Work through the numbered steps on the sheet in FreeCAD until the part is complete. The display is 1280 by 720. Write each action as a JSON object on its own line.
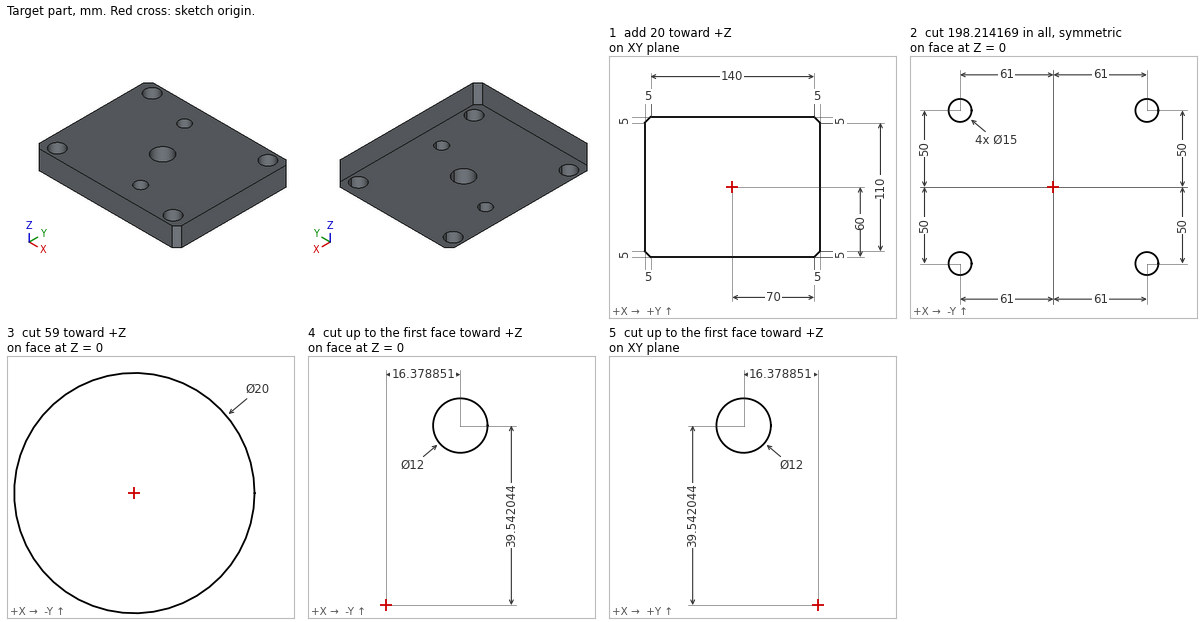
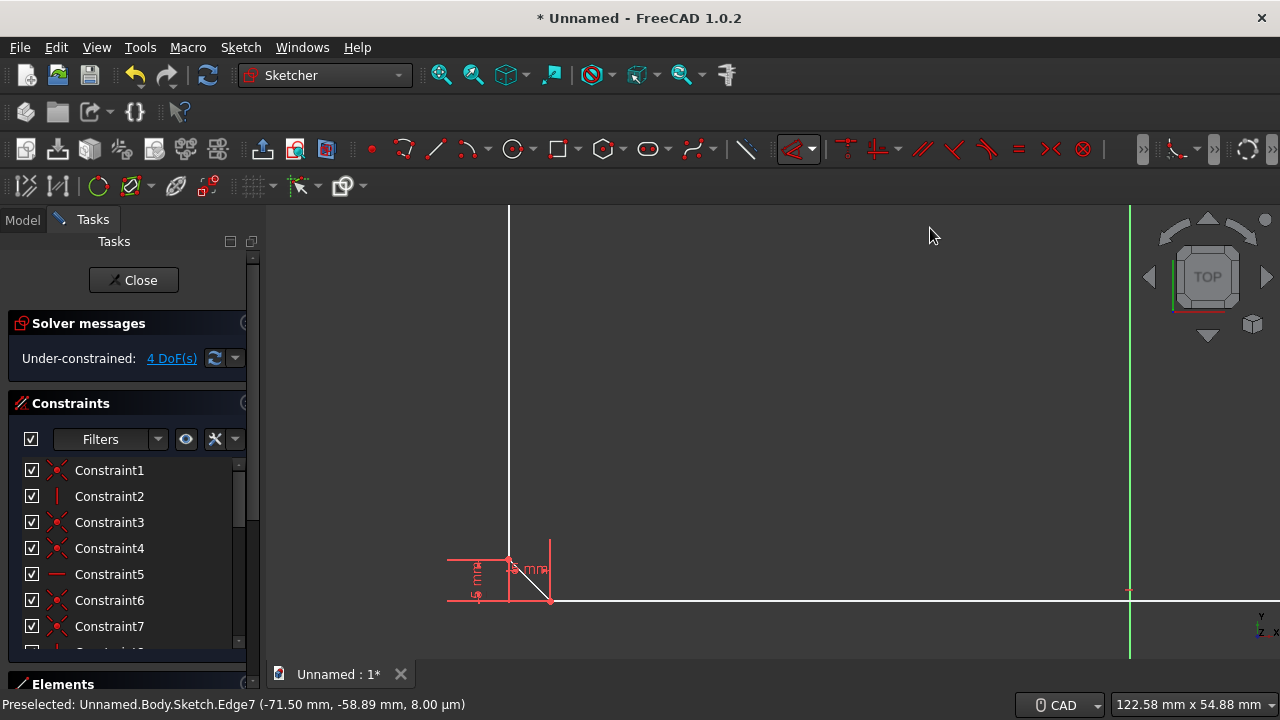
{"action": "scroll", "coordinate": [521, 574], "scroll_direction": "down", "scroll_amount": 6}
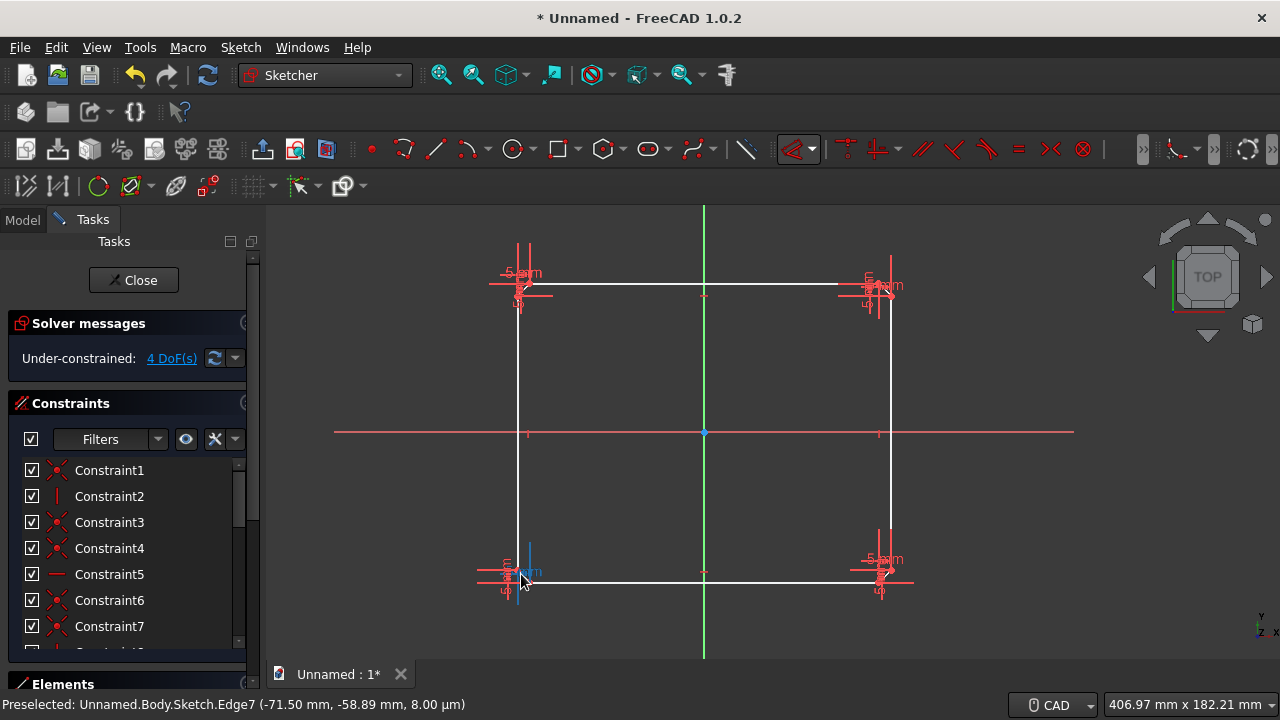
{"action": "left_click", "coordinate": [891, 488]}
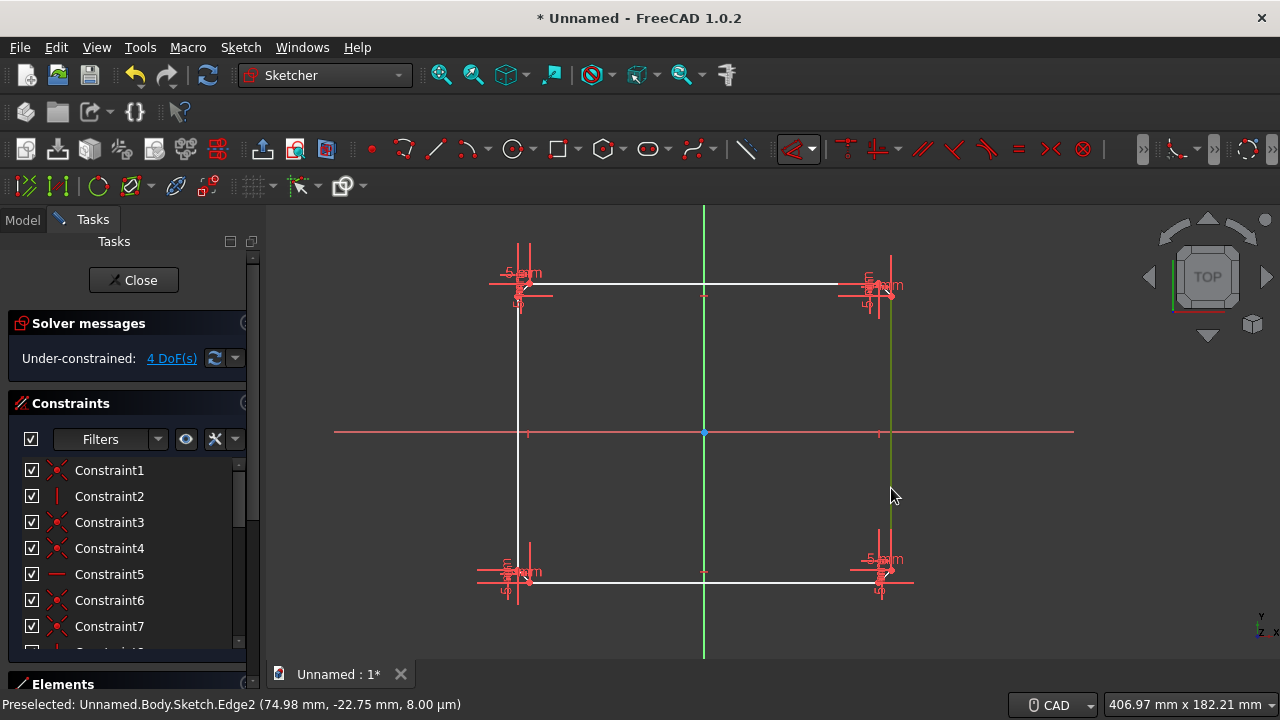
{"action": "key", "text": "i"}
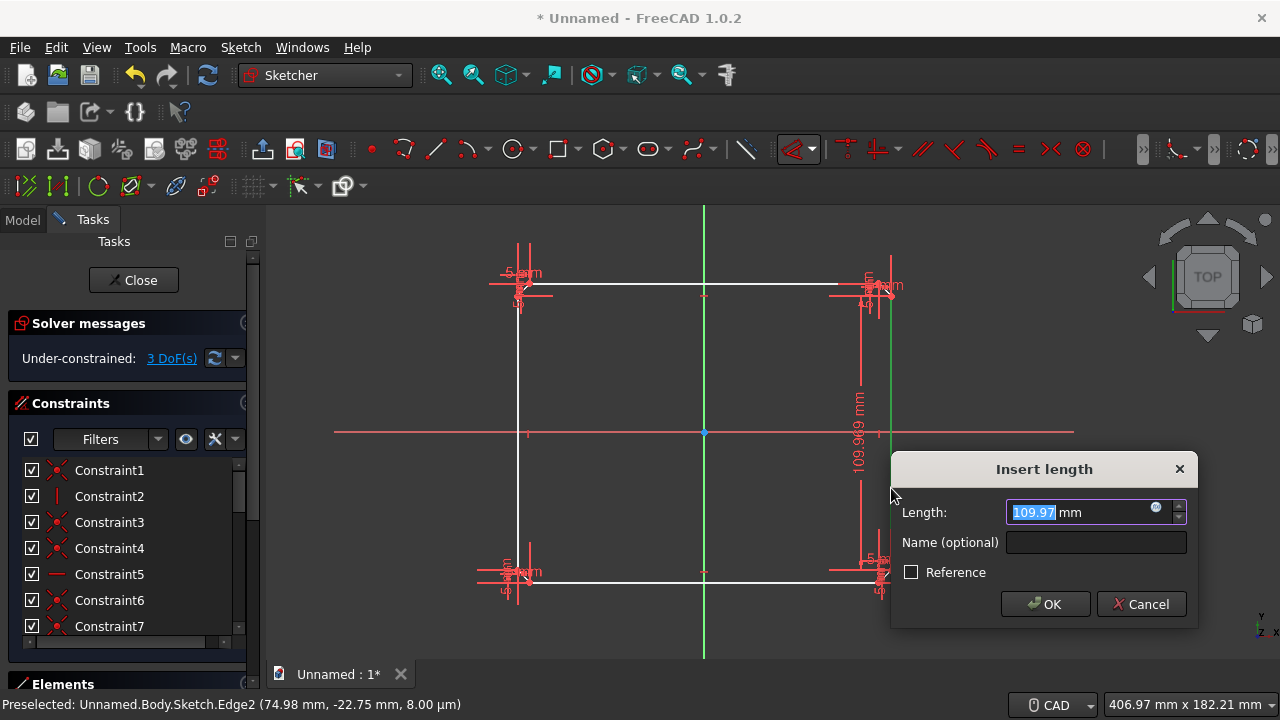
{"action": "type", "text": "110"}
{"action": "key", "text": "Return"}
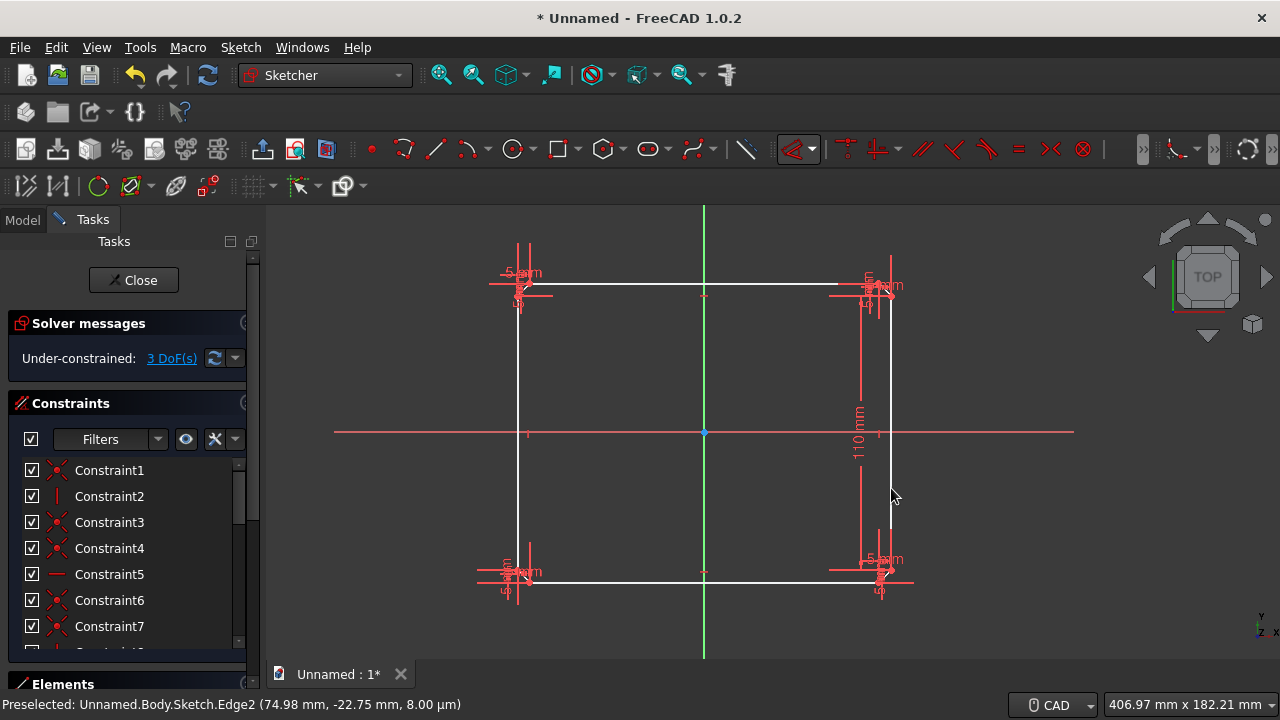
{"action": "left_click", "coordinate": [774, 284]}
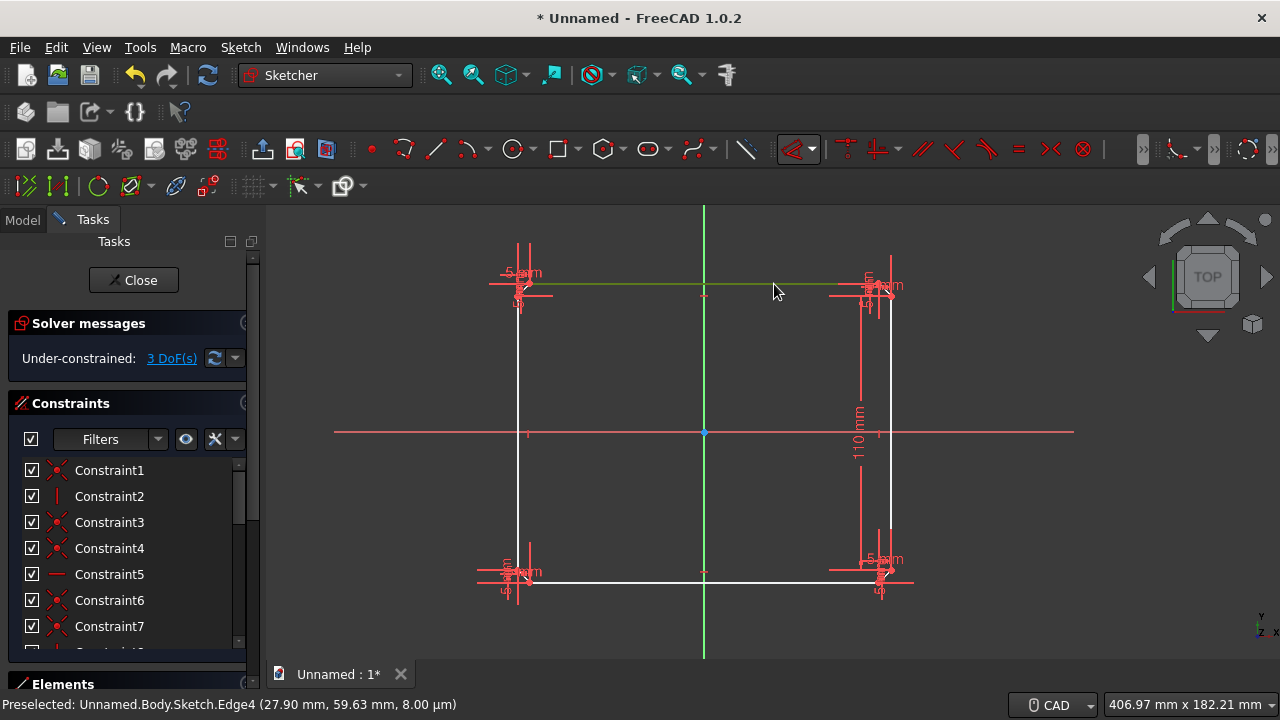
{"action": "left_click", "coordinate": [814, 150]}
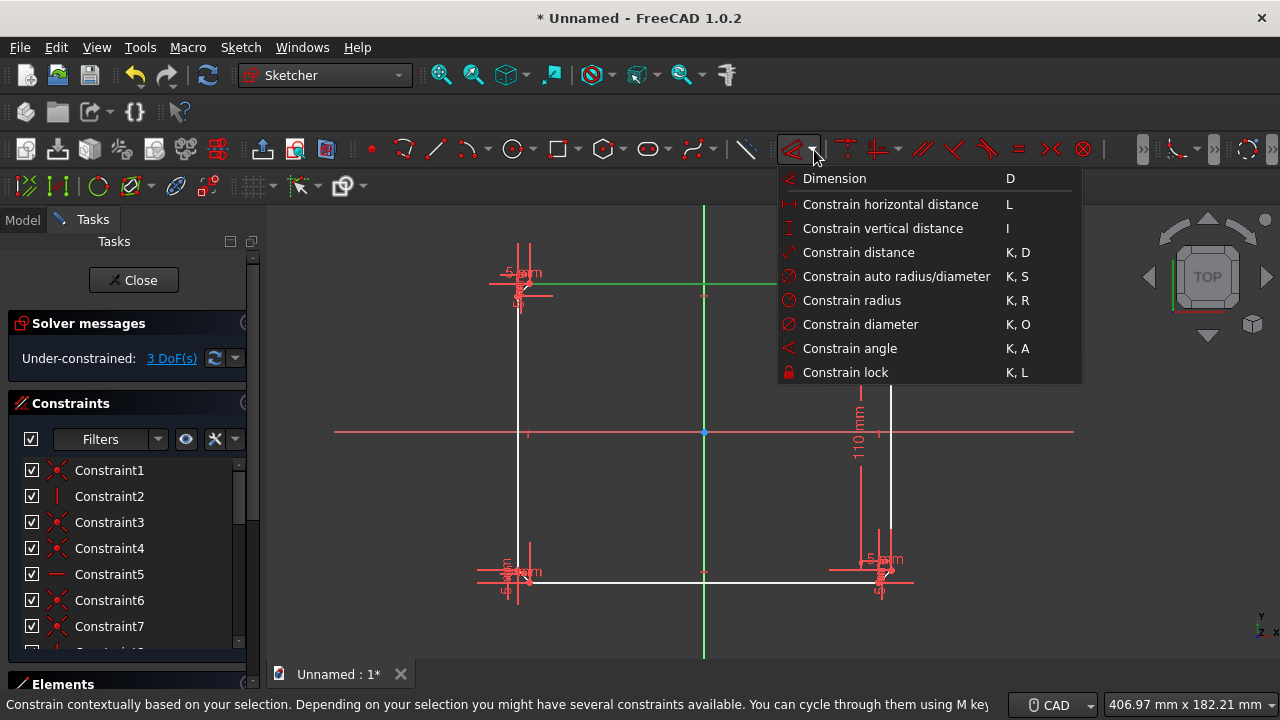
{"action": "left_click", "coordinate": [930, 204]}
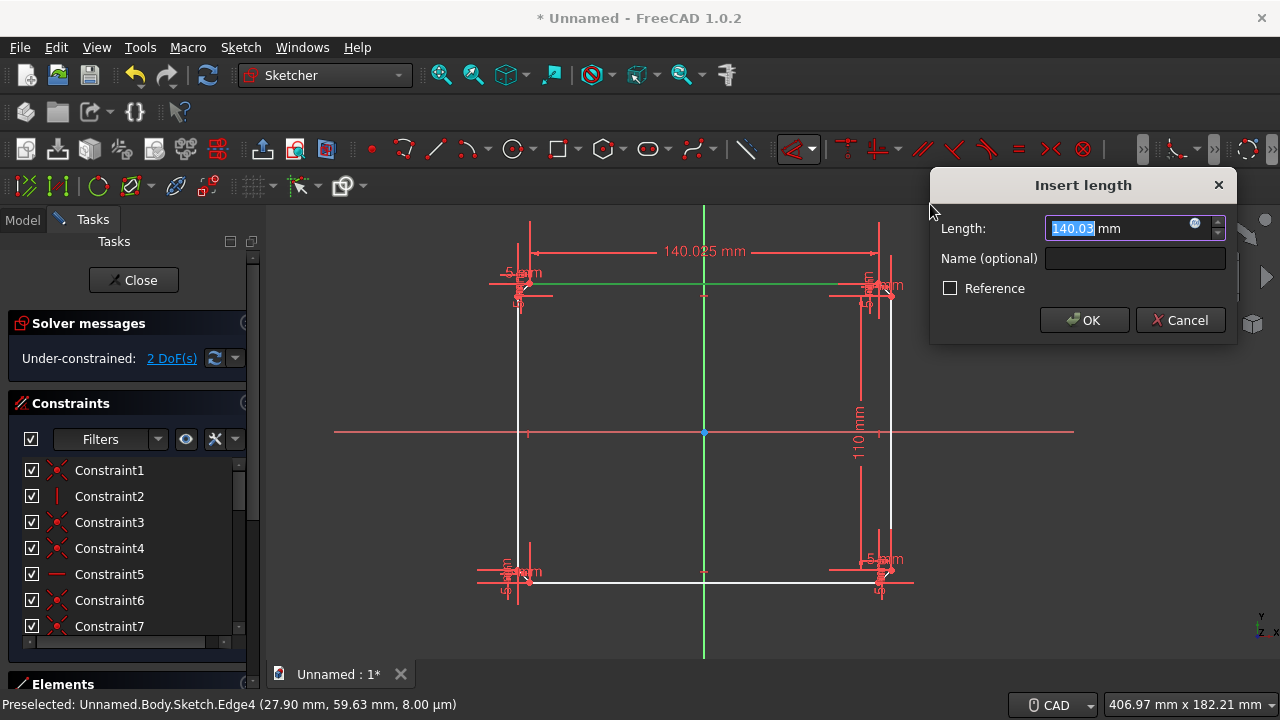
{"action": "type", "text": "140"}
{"action": "key", "text": "Return"}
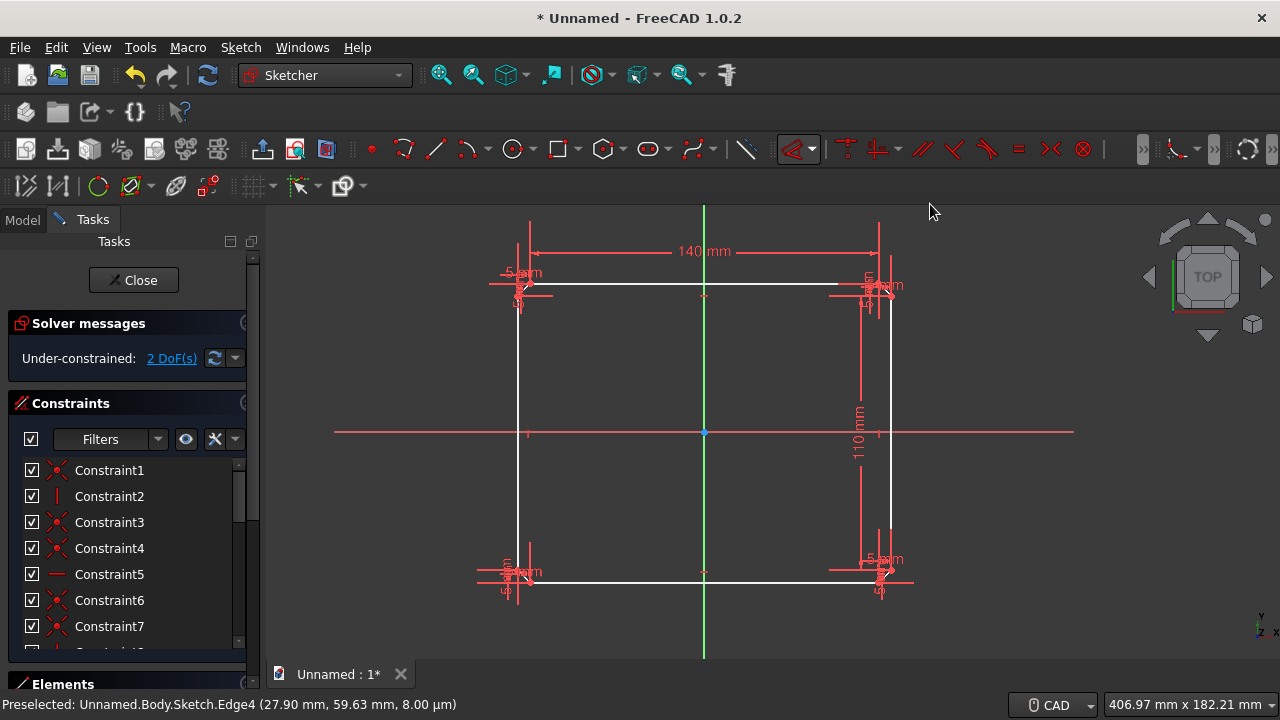
{"action": "left_click", "coordinate": [879, 583]}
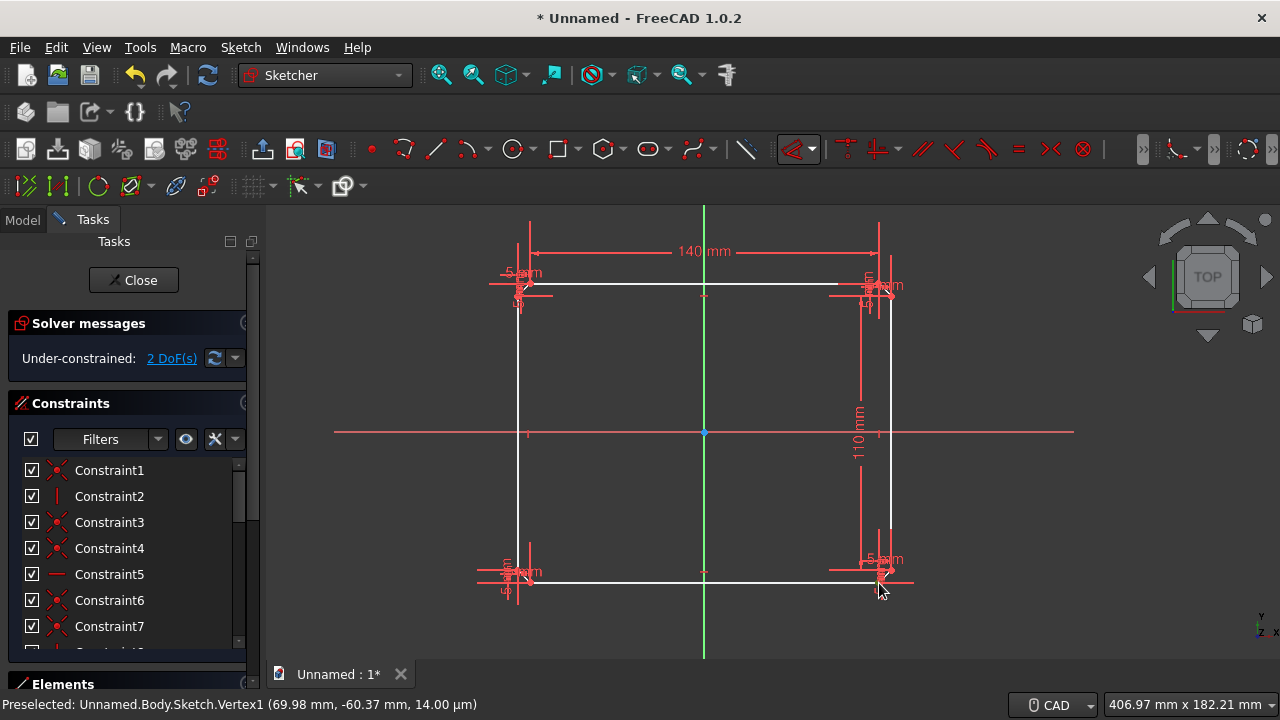
{"action": "left_click", "coordinate": [814, 150]}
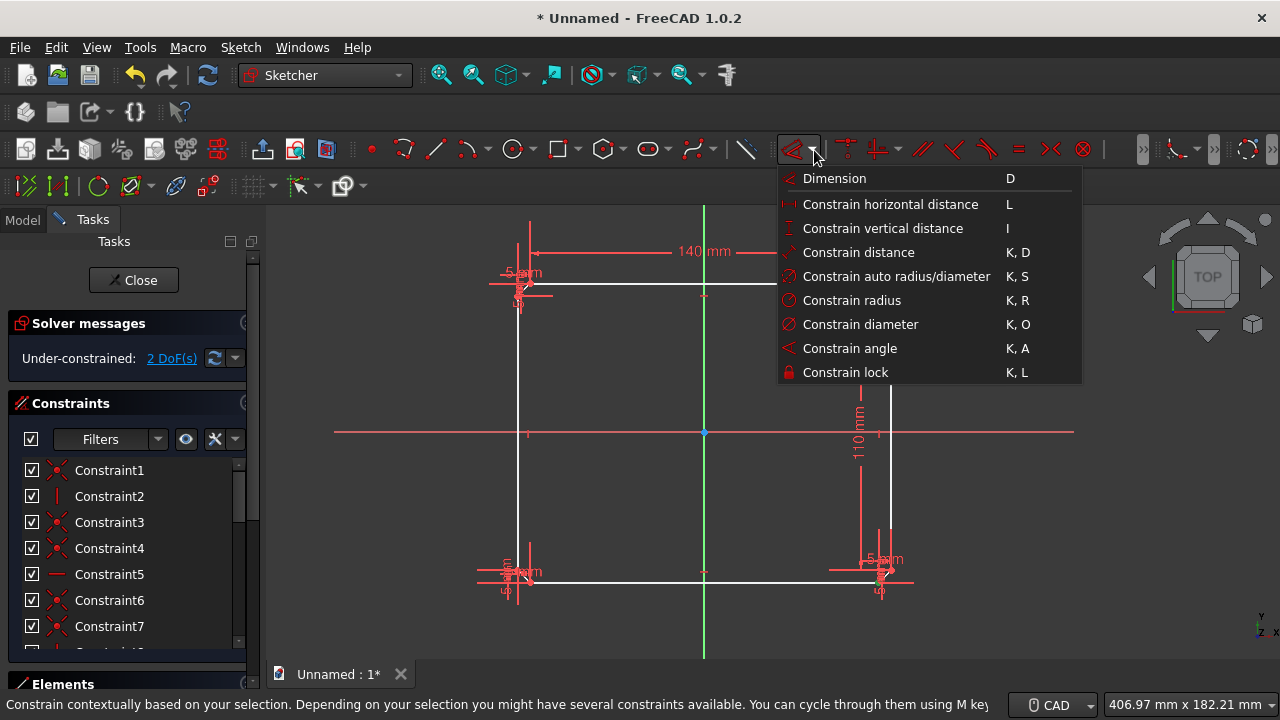
{"action": "left_click", "coordinate": [930, 204]}